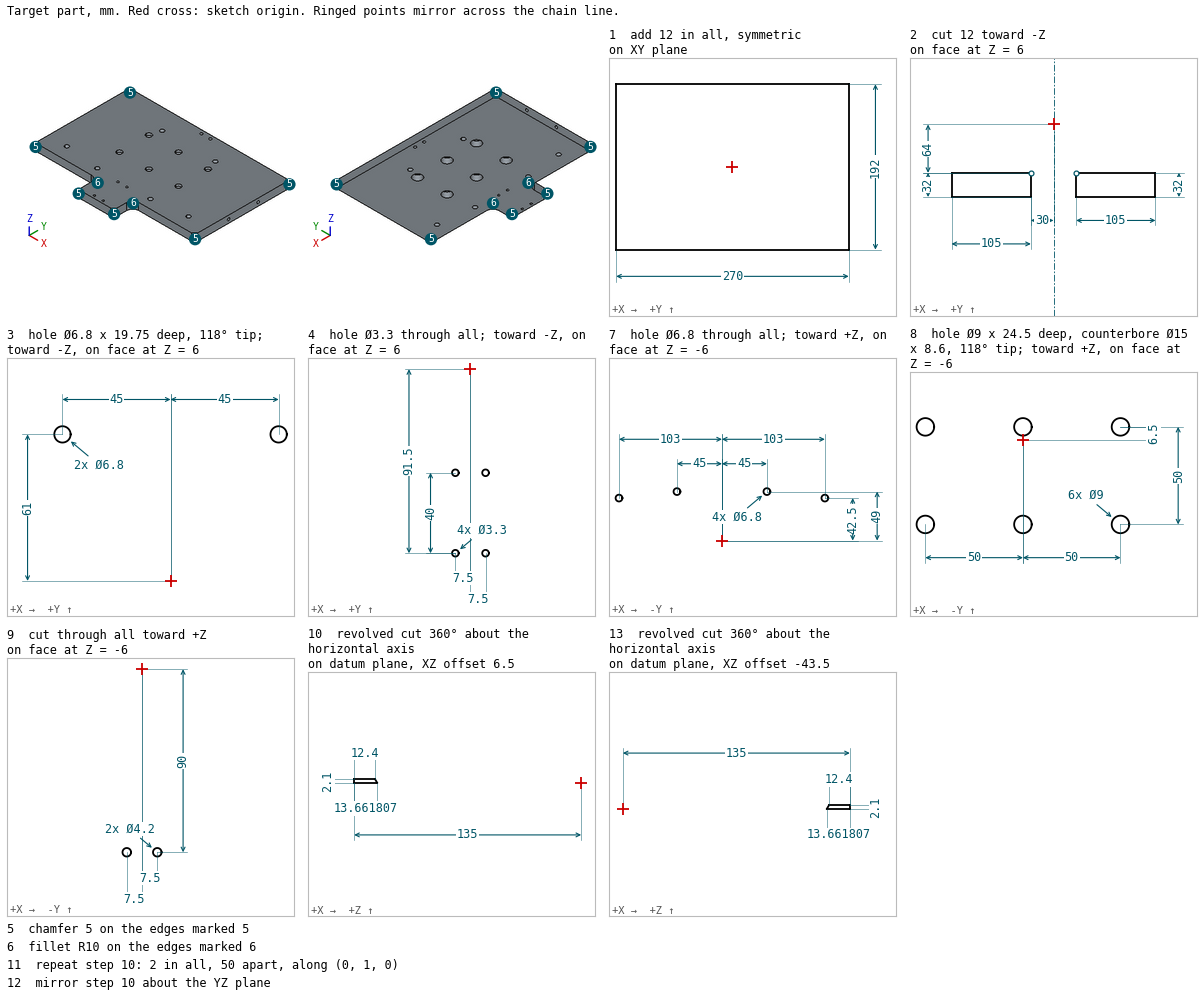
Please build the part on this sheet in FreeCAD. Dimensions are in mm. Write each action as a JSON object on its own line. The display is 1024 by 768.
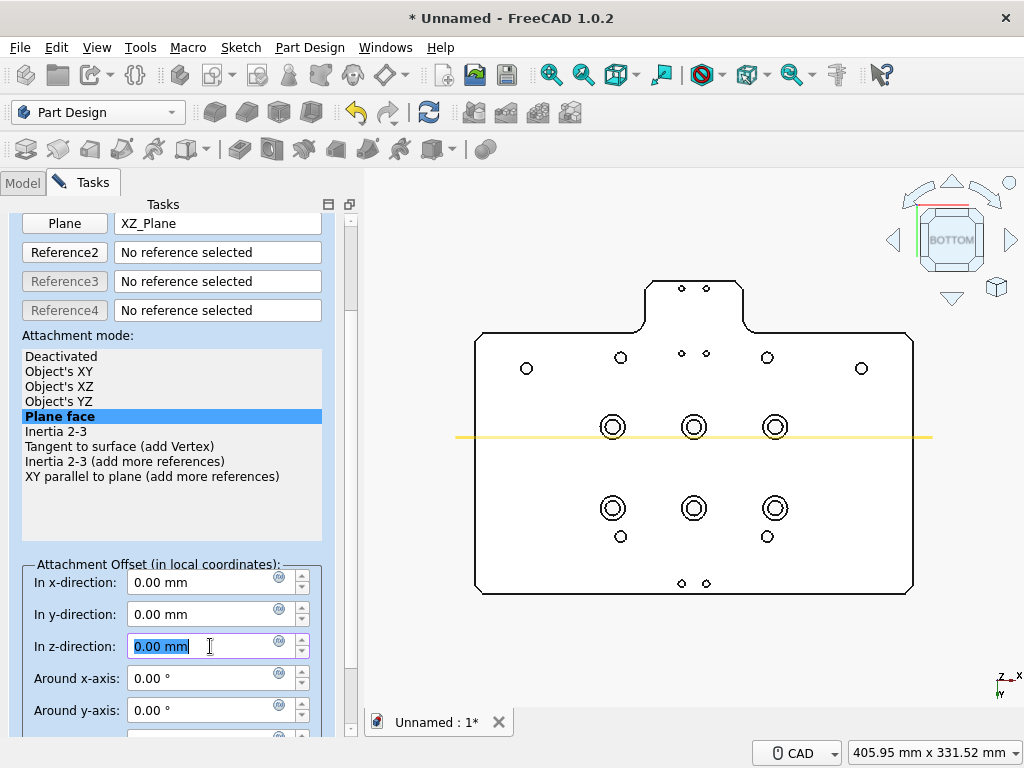
{"action": "type", "text": "-43.5"}
{"action": "key", "text": "Tab"}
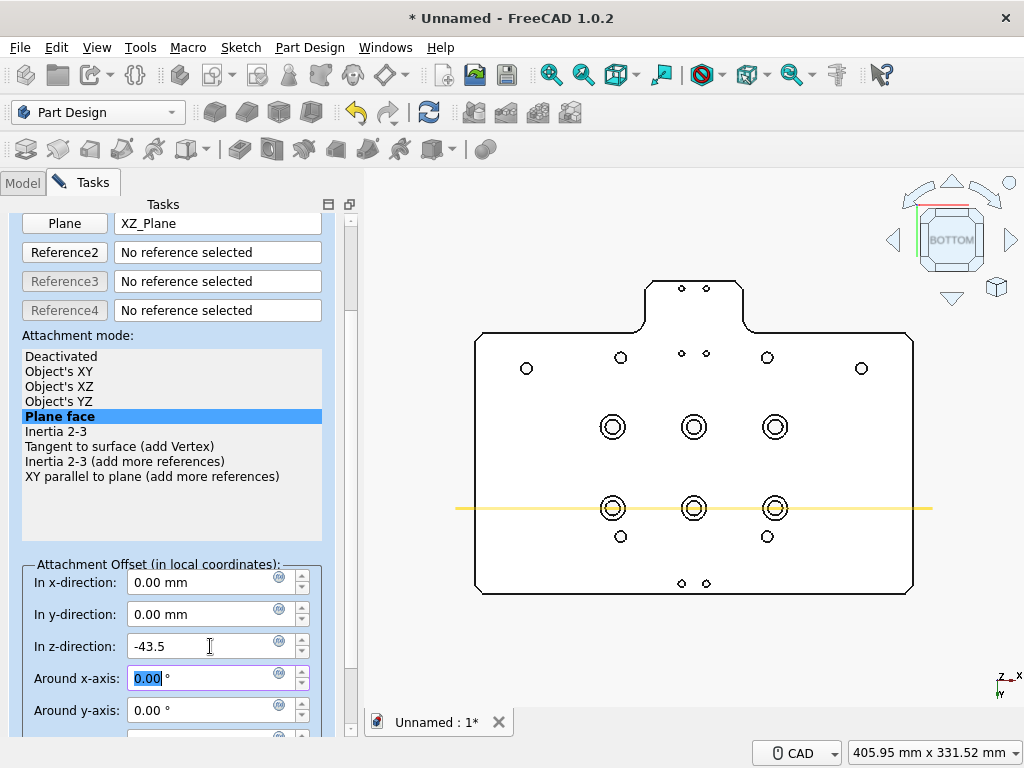
{"action": "scroll", "coordinate": [351, 475], "scroll_direction": "up", "scroll_amount": 3}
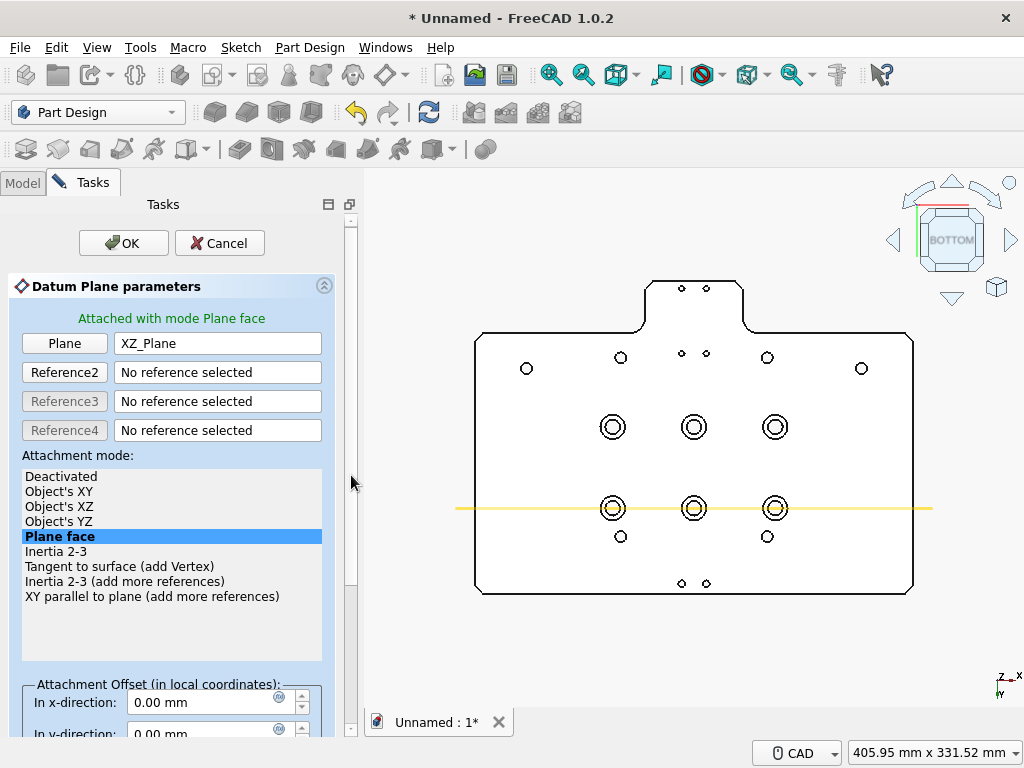
{"action": "left_click", "coordinate": [124, 243]}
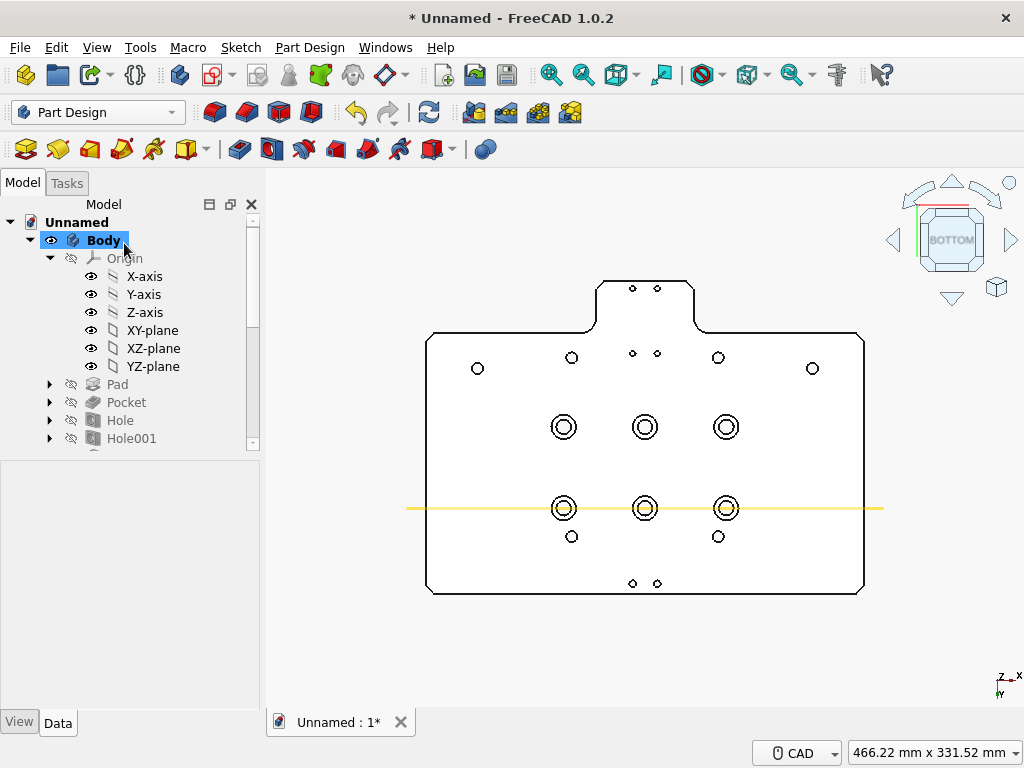
{"action": "scroll", "coordinate": [100, 326], "scroll_direction": "down", "scroll_amount": 3}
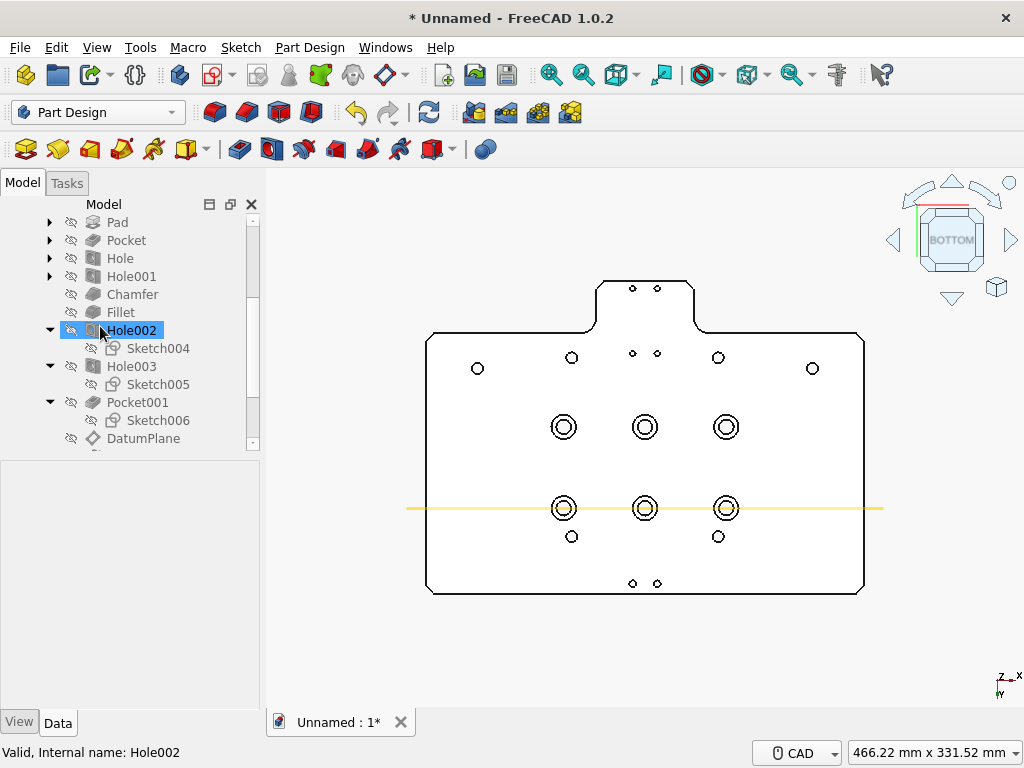
{"action": "scroll", "coordinate": [140, 326], "scroll_direction": "up", "scroll_amount": 15}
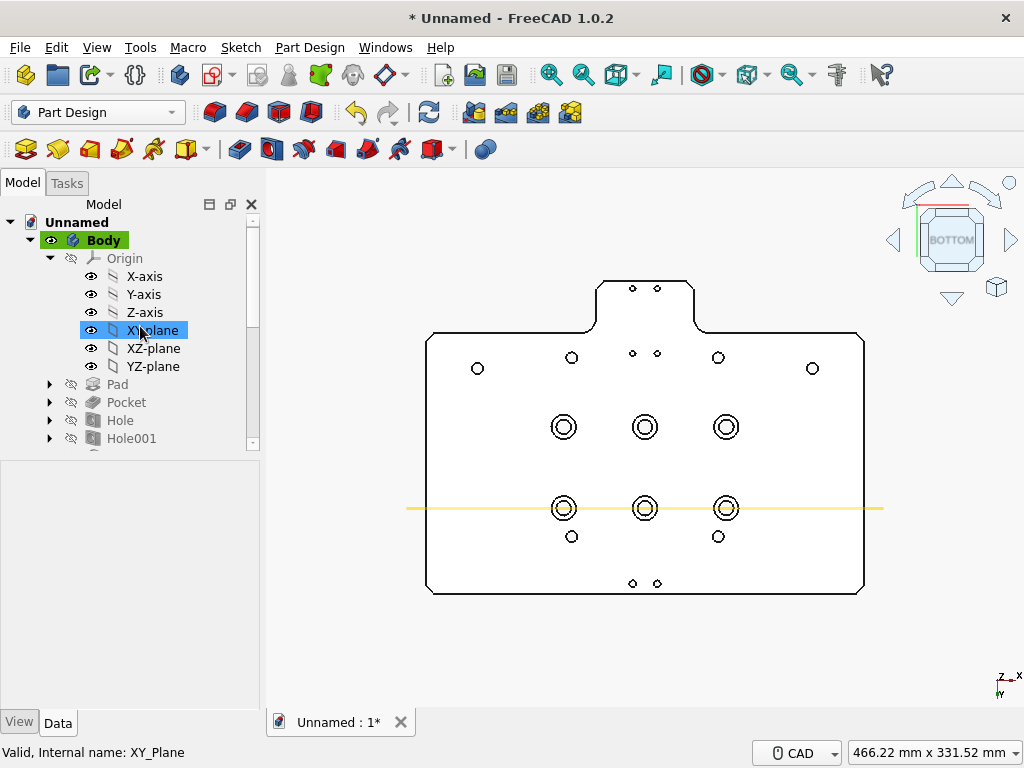
{"action": "scroll", "coordinate": [100, 326], "scroll_direction": "down", "scroll_amount": 6}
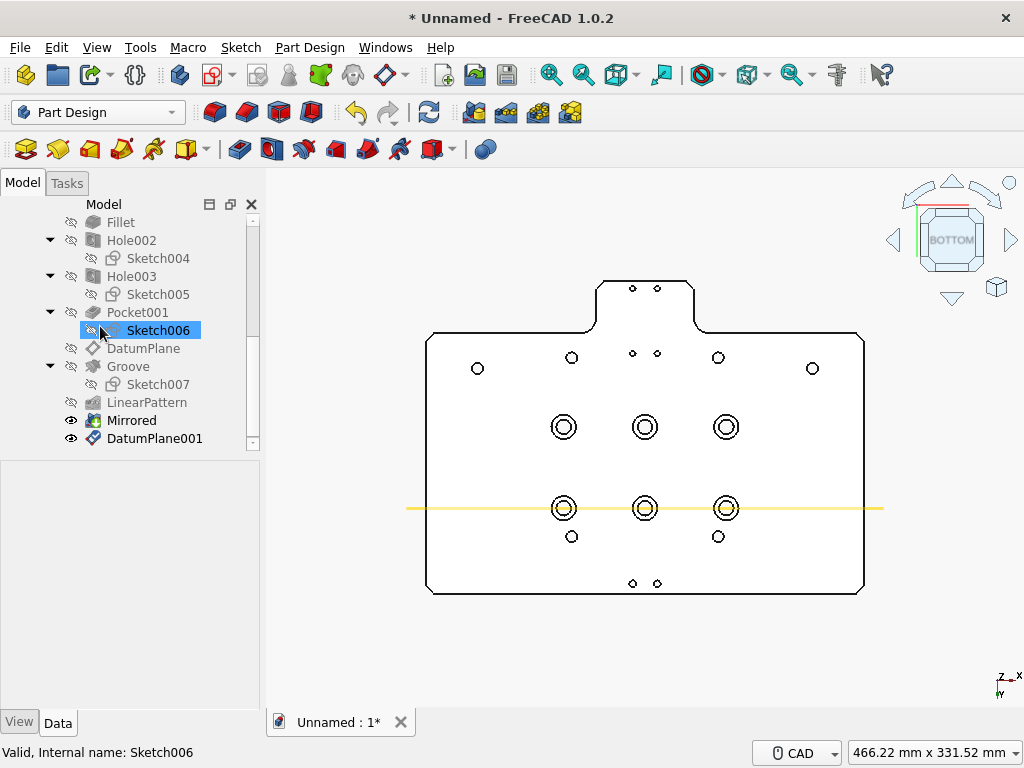
{"action": "left_click", "coordinate": [116, 438]}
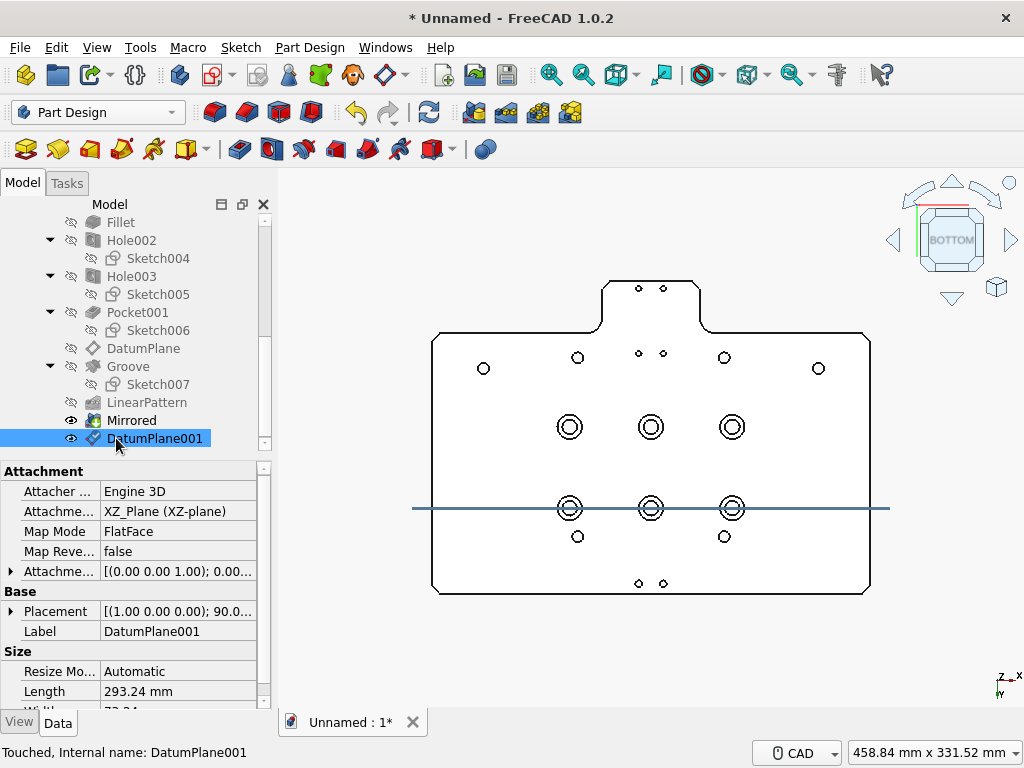
{"action": "left_click", "coordinate": [212, 76]}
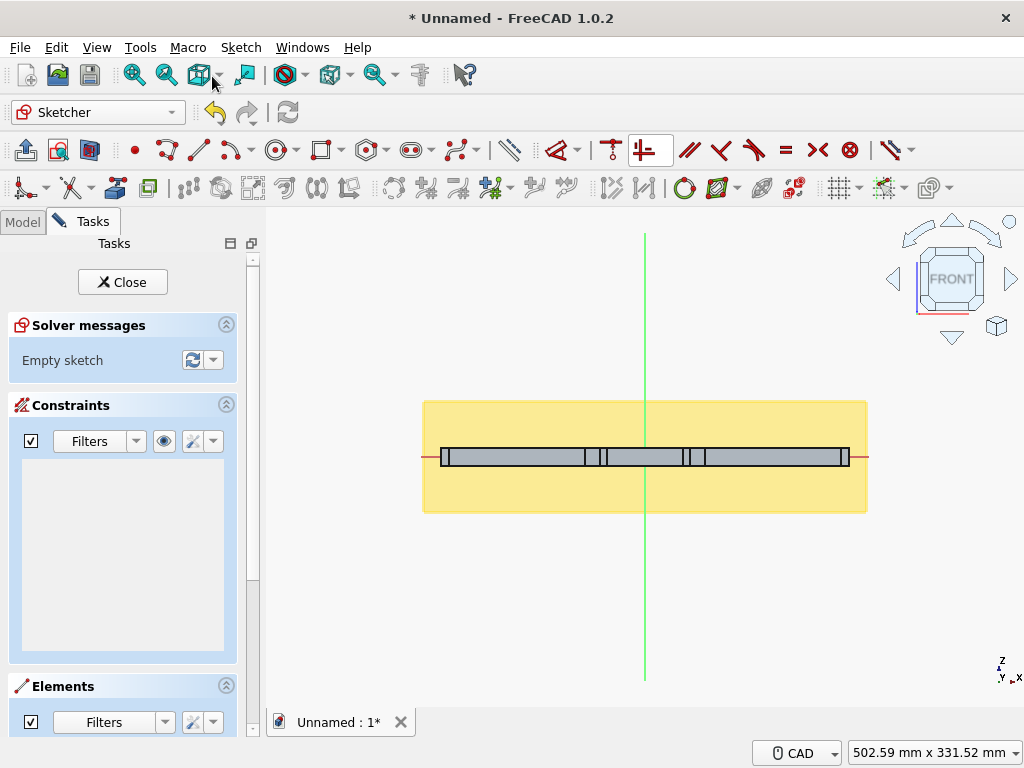
{"action": "left_click", "coordinate": [90, 150]}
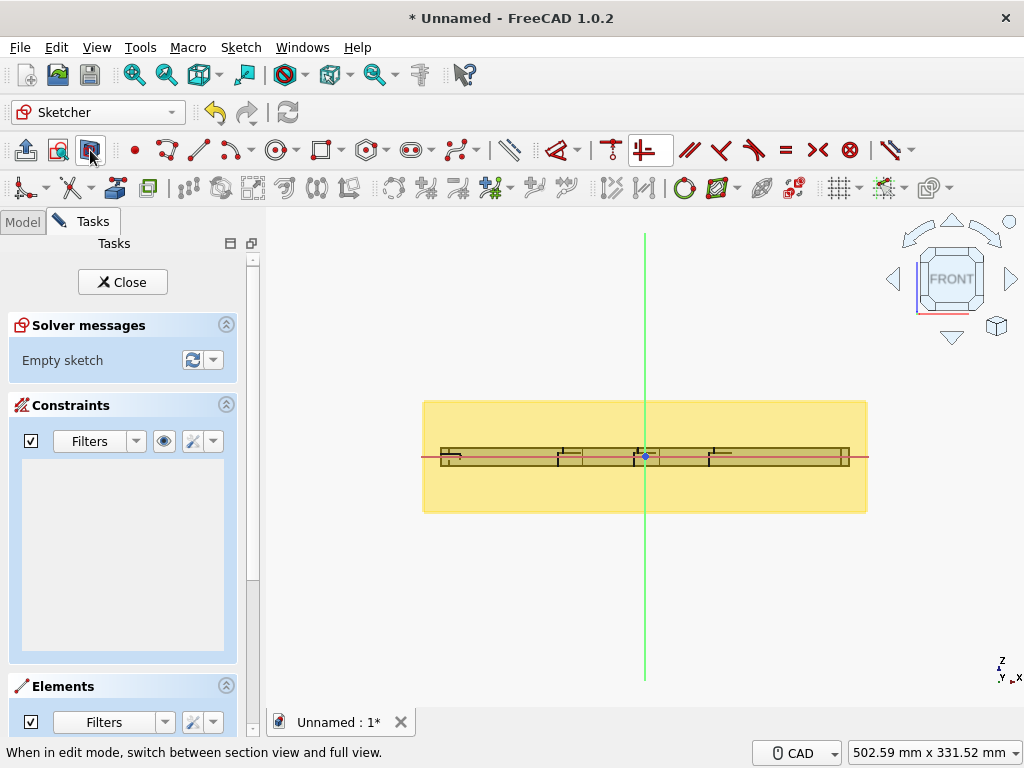
{"action": "scroll", "coordinate": [852, 455], "scroll_direction": "up", "scroll_amount": 15}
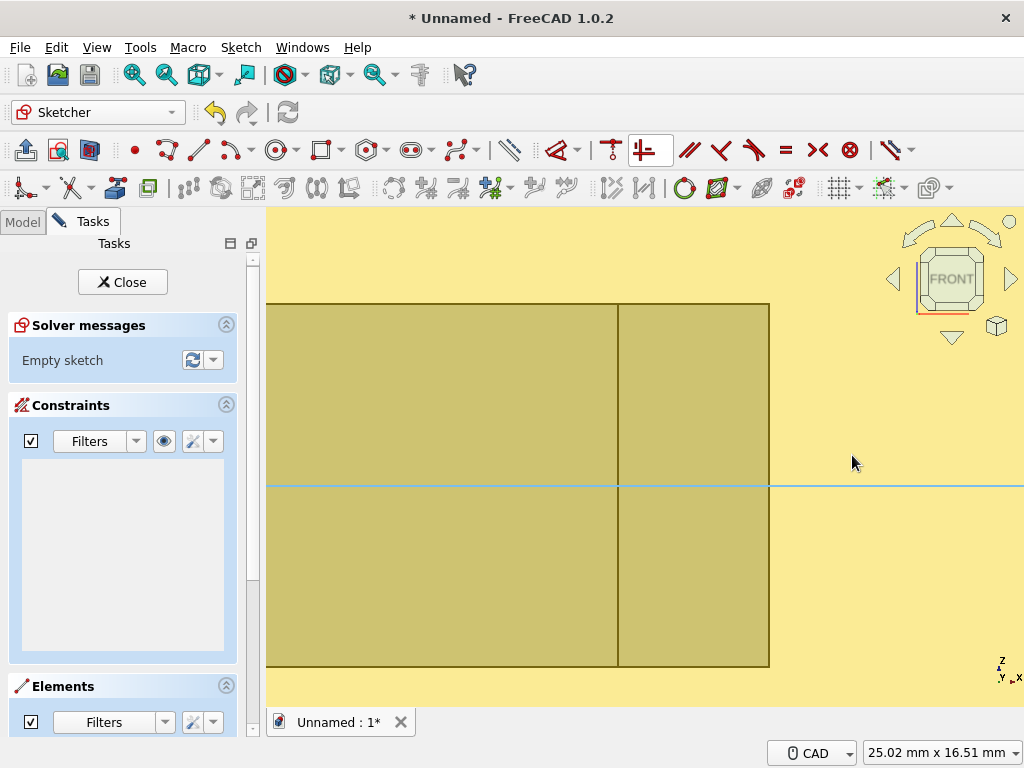
{"action": "left_click", "coordinate": [168, 150]}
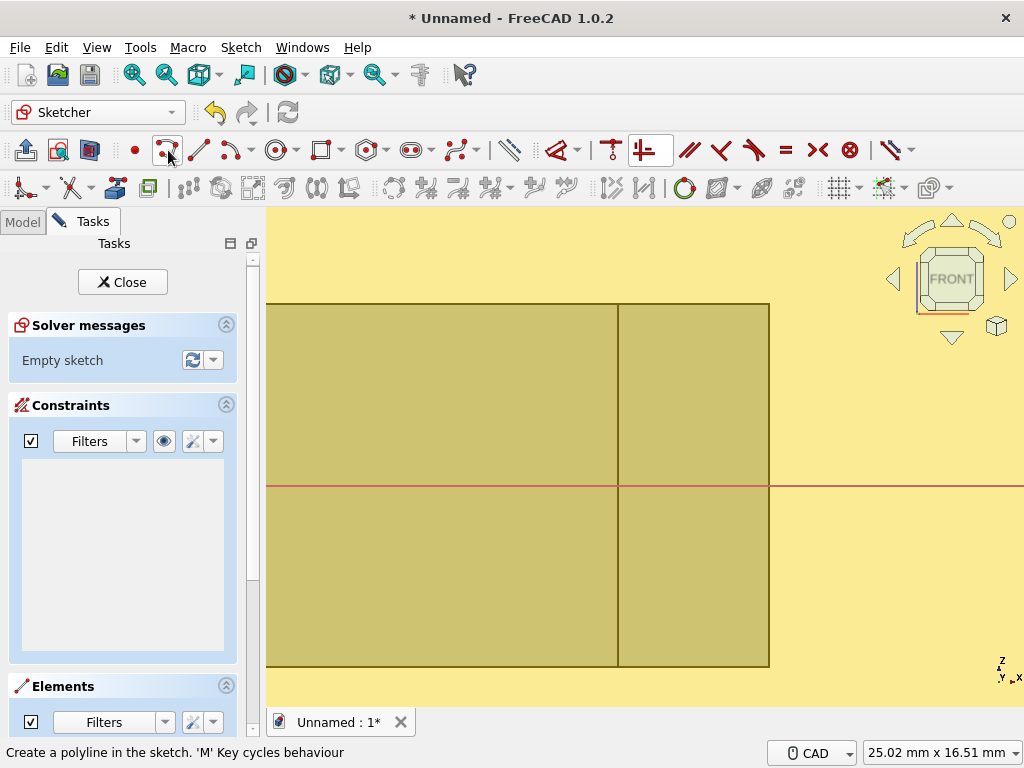
{"action": "left_click", "coordinate": [355, 486]}
{"action": "left_click", "coordinate": [393, 422]}
{"action": "left_click", "coordinate": [769, 422]}
{"action": "left_click", "coordinate": [769, 477]}
{"action": "left_click", "coordinate": [355, 486]}
{"action": "key", "text": "Escape"}
{"action": "key", "text": "Escape"}